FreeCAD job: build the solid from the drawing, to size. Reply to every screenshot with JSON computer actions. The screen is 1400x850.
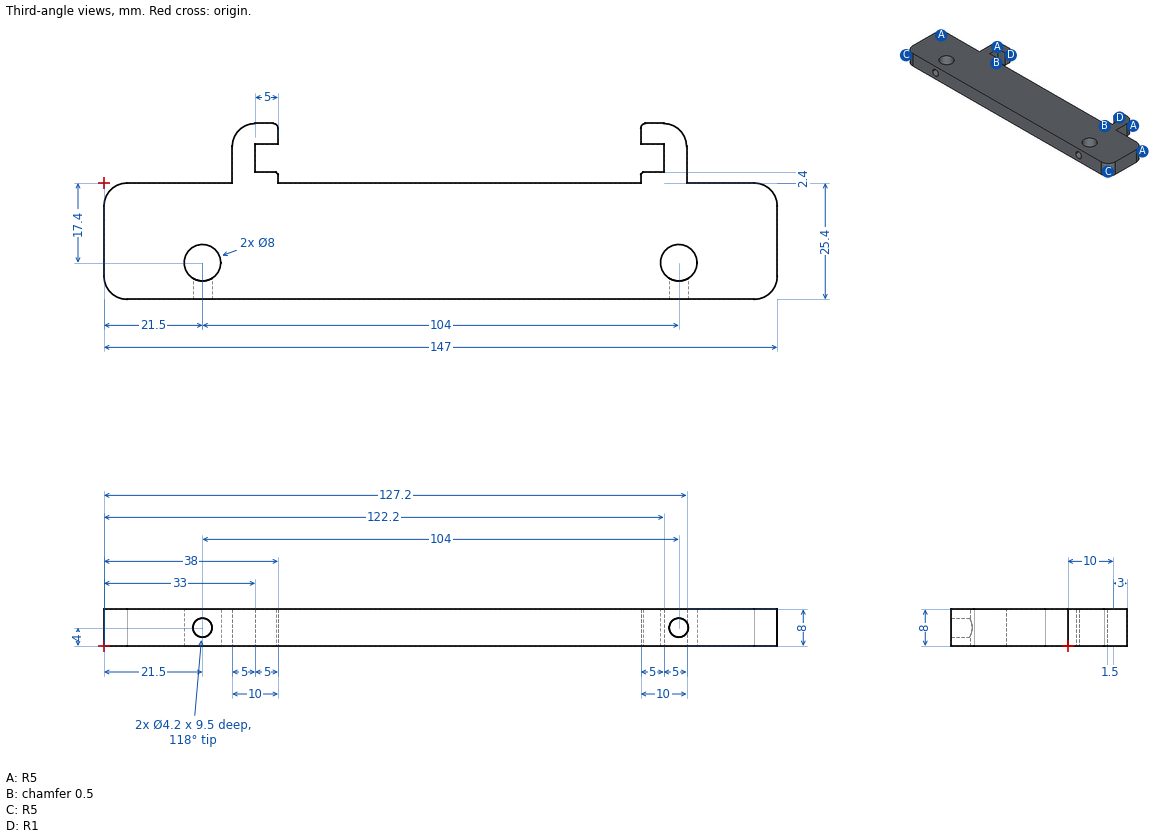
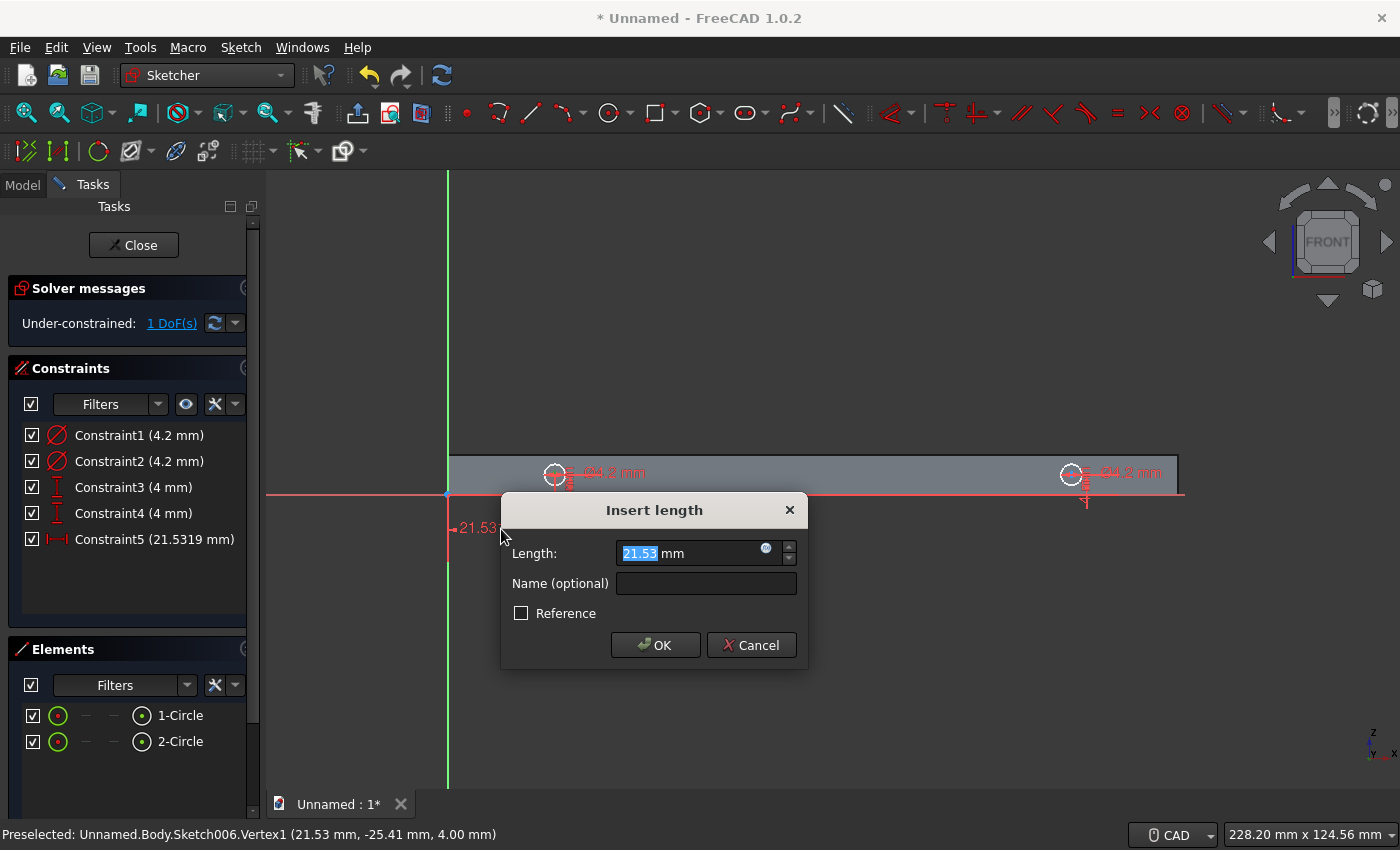
{"action": "type", "text": "21.5"}
{"action": "key", "text": "Return"}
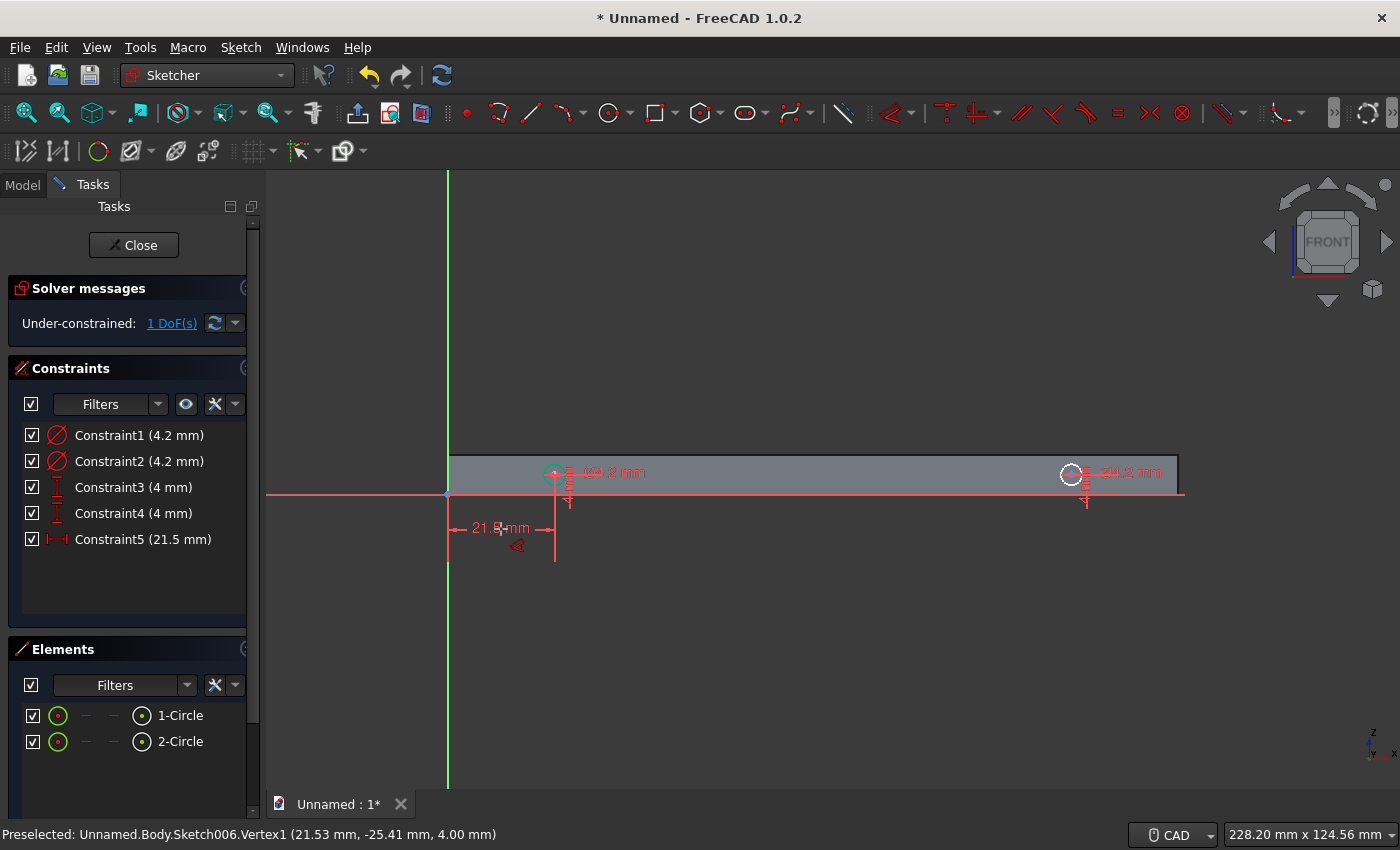
{"action": "left_click", "coordinate": [555, 475]}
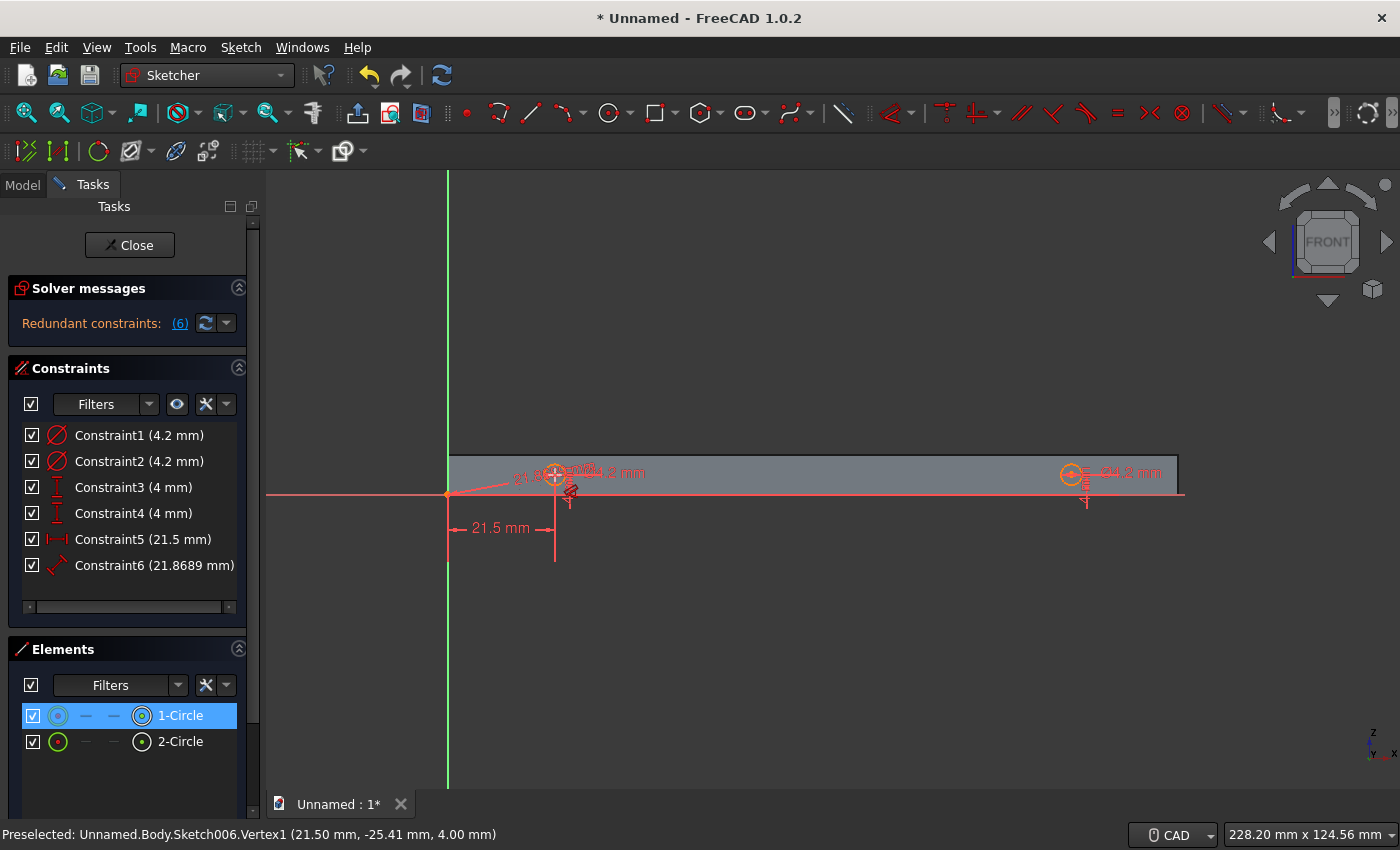
{"action": "left_click", "coordinate": [1071, 475]}
{"action": "left_click", "coordinate": [813, 441]}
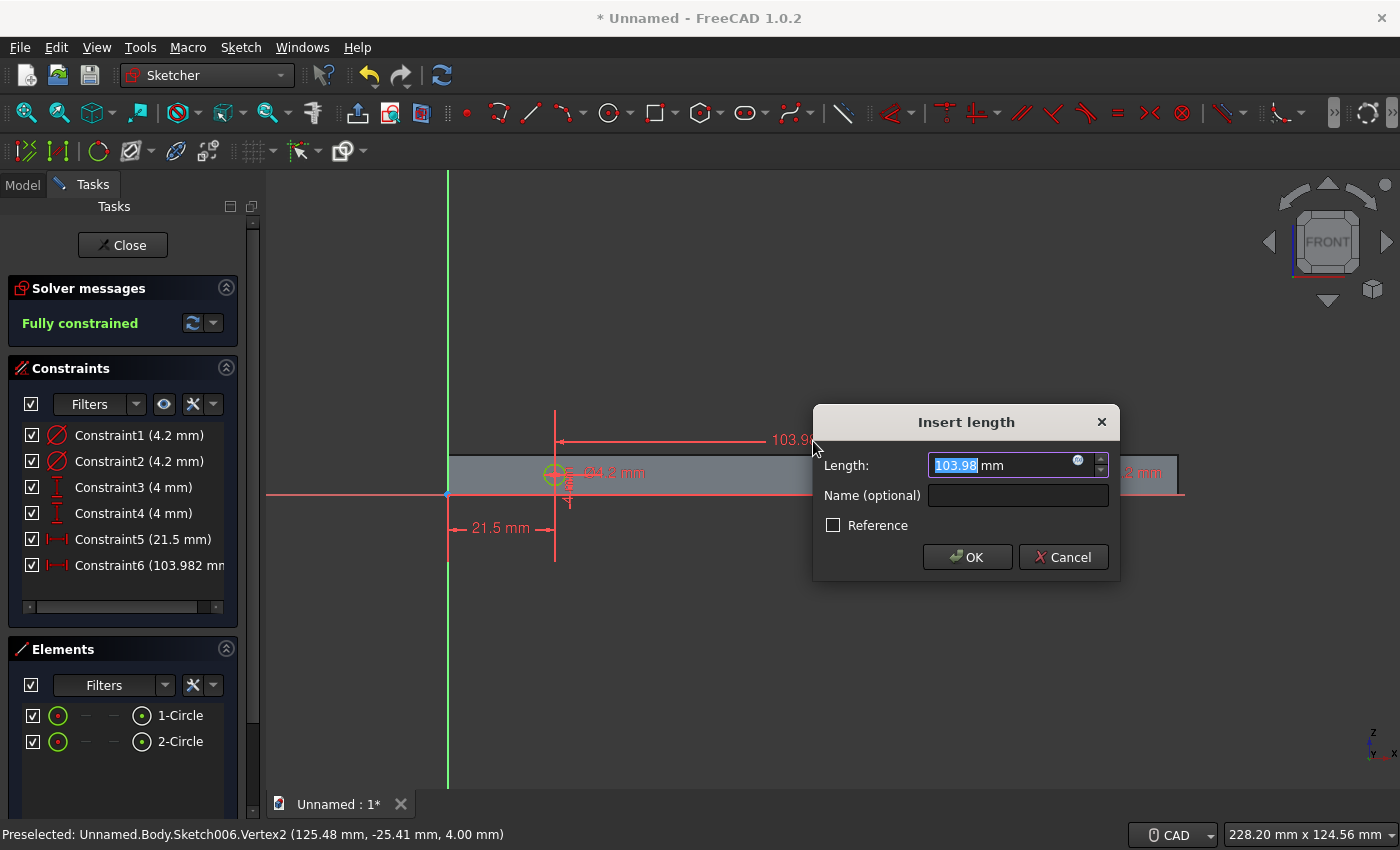
{"action": "type", "text": "104"}
{"action": "key", "text": "Return"}
{"action": "key", "text": "Escape"}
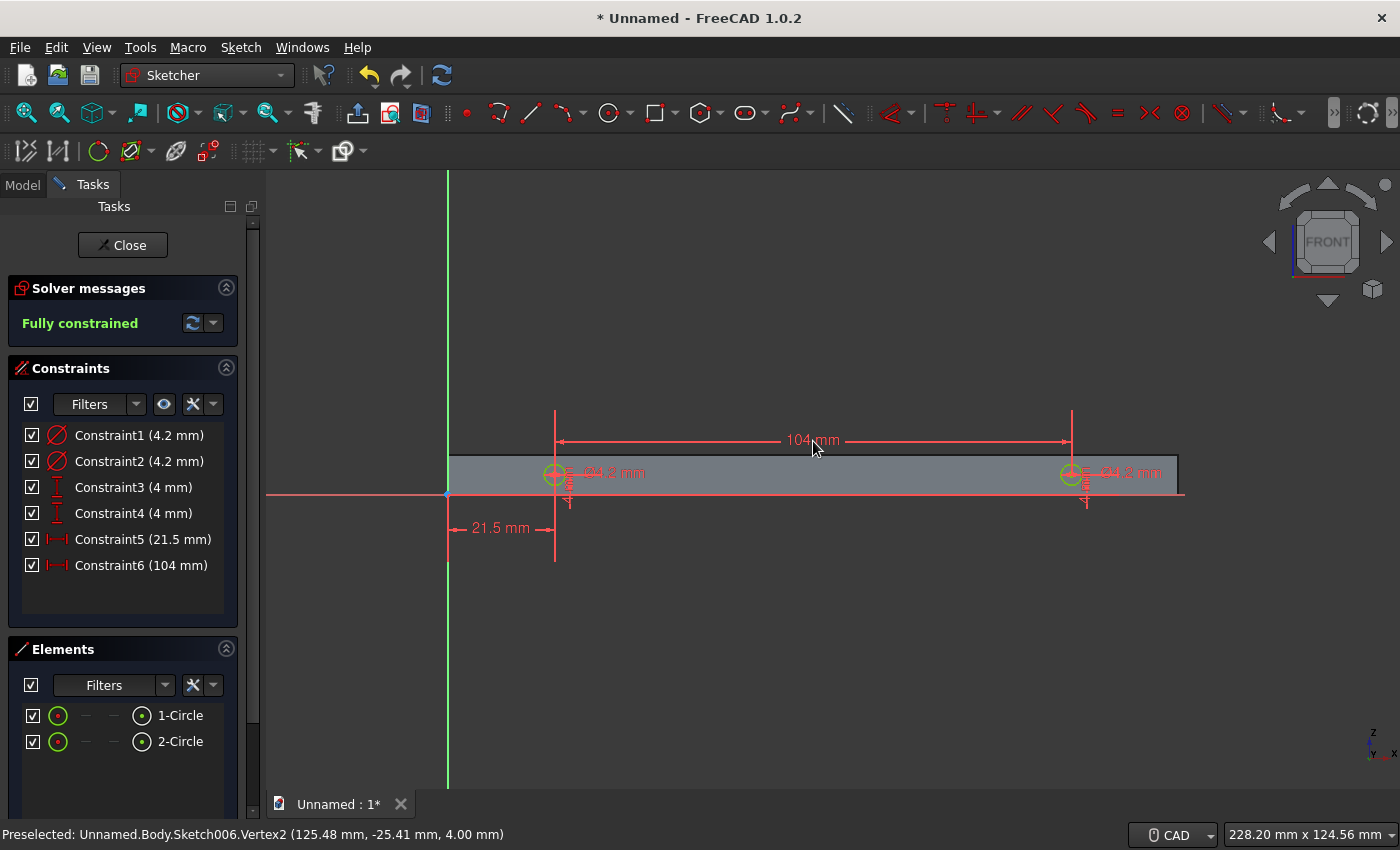
{"action": "left_click", "coordinate": [123, 245]}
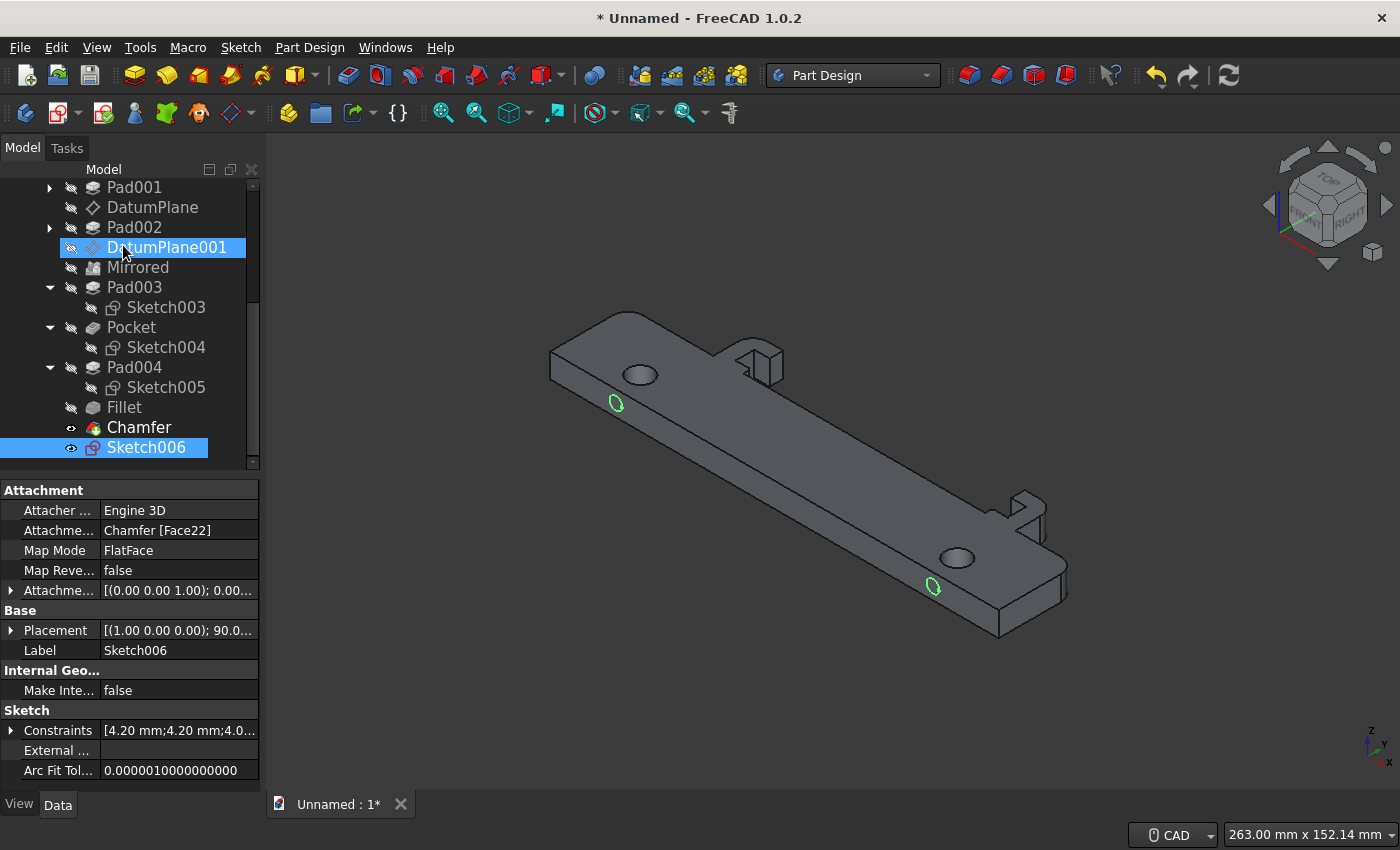
{"action": "left_click", "coordinate": [382, 76]}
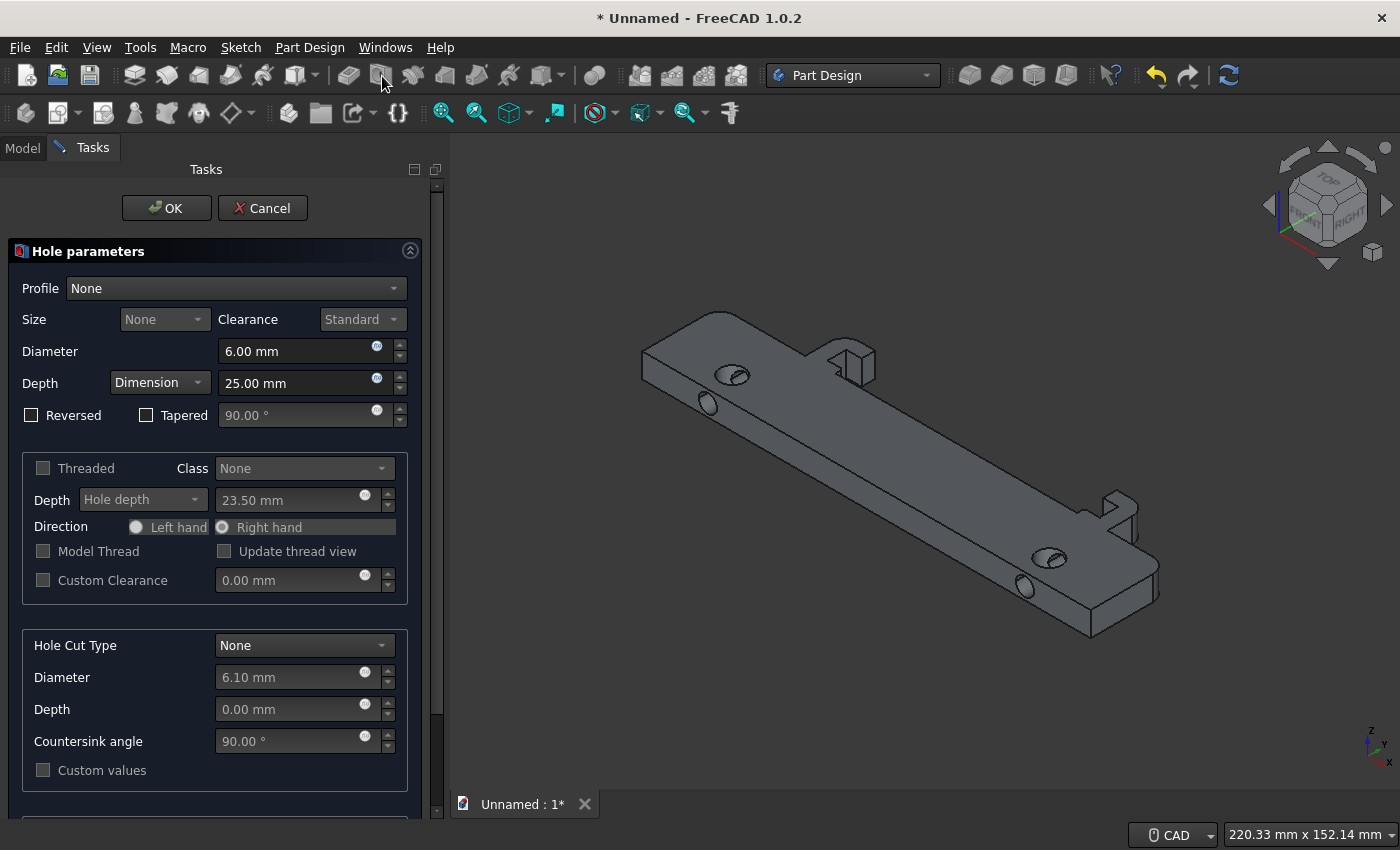
{"action": "triple_click", "coordinate": [305, 351]}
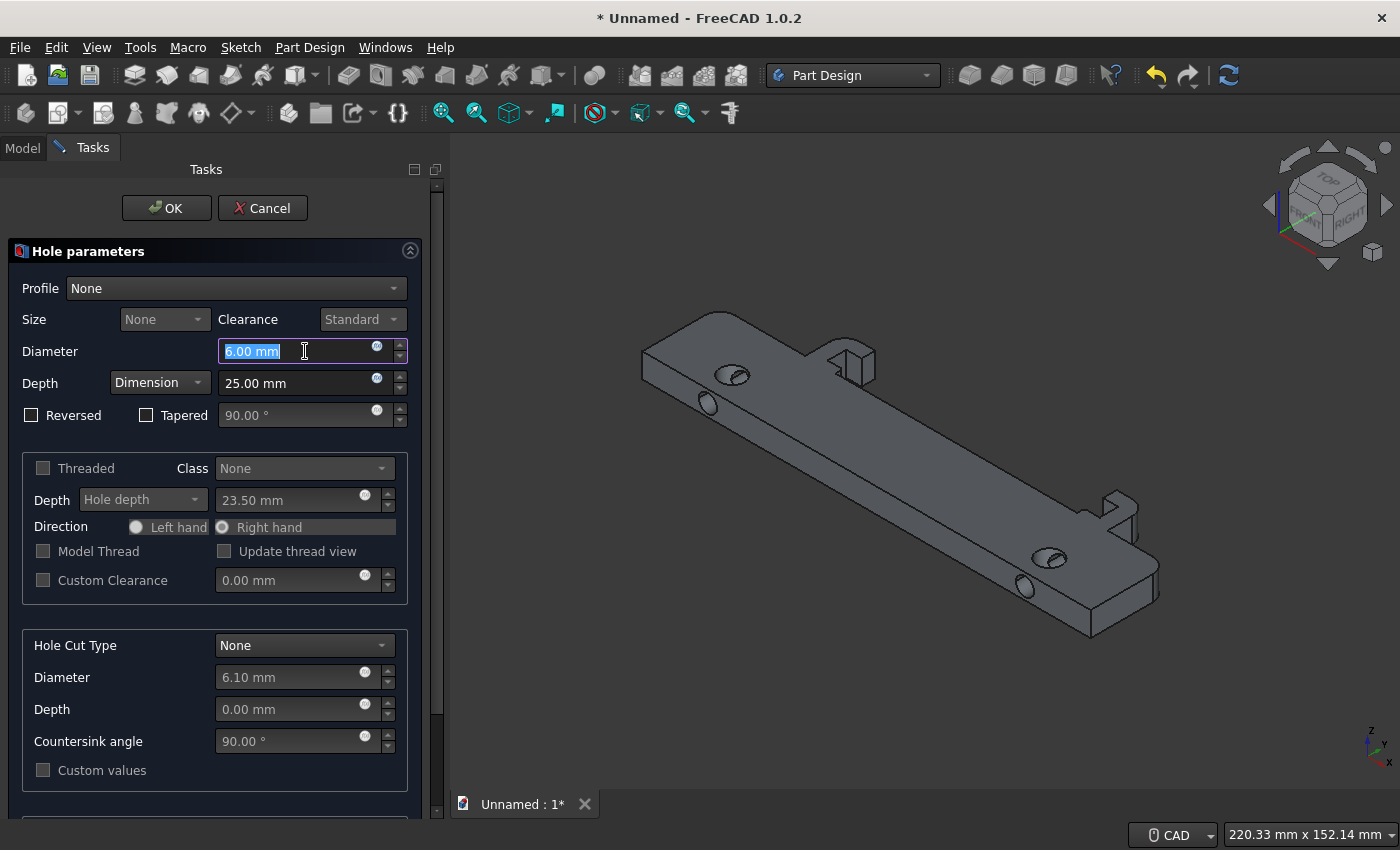
{"action": "type", "text": "4.2"}
{"action": "key", "text": "Tab"}